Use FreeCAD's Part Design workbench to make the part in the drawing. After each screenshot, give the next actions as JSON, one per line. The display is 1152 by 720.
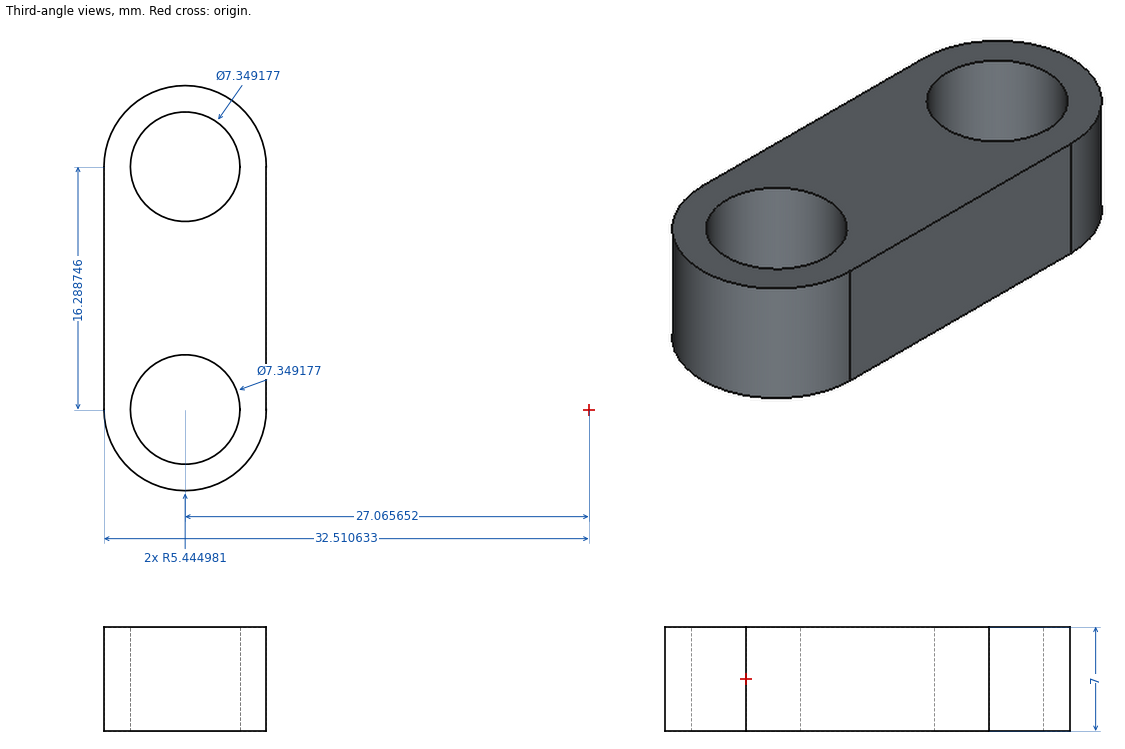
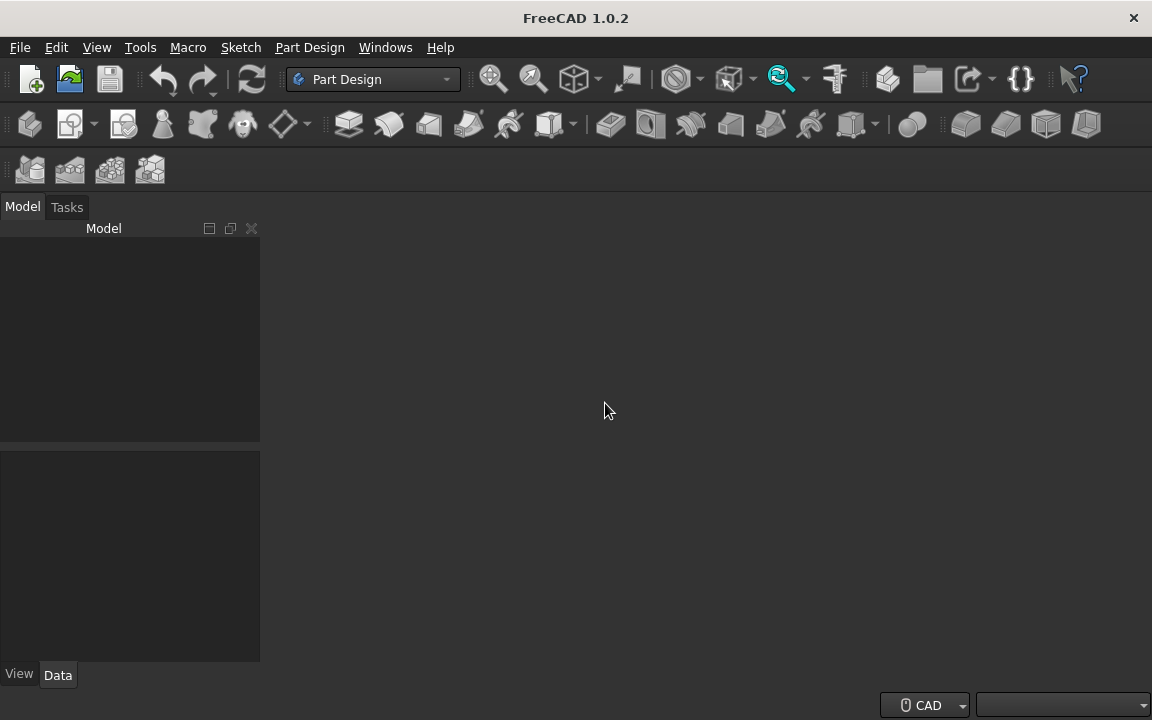
{"action": "left_click", "coordinate": [30, 80]}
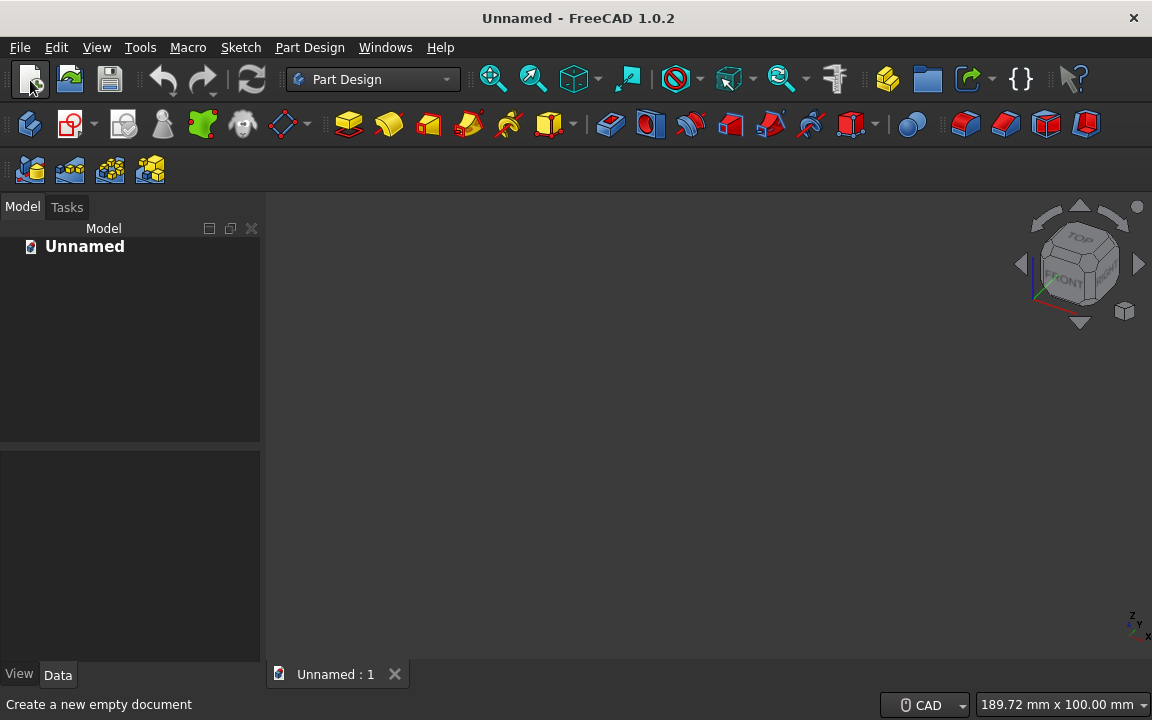
{"action": "left_click", "coordinate": [70, 124]}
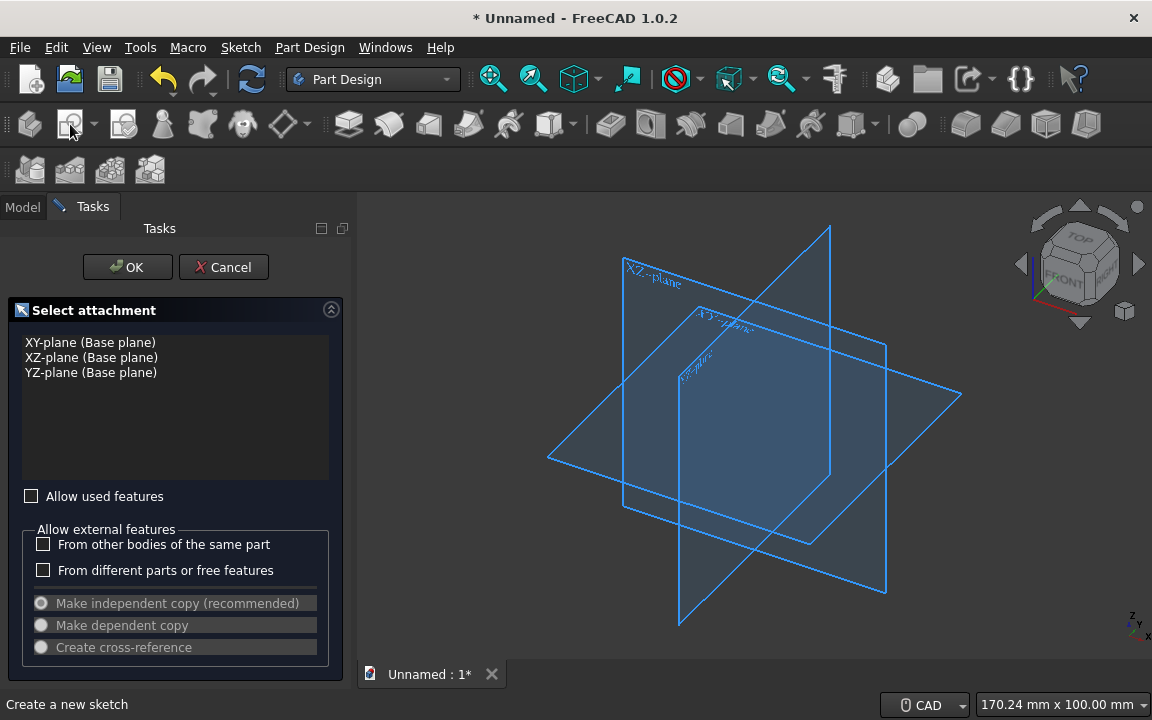
{"action": "left_click", "coordinate": [82, 342]}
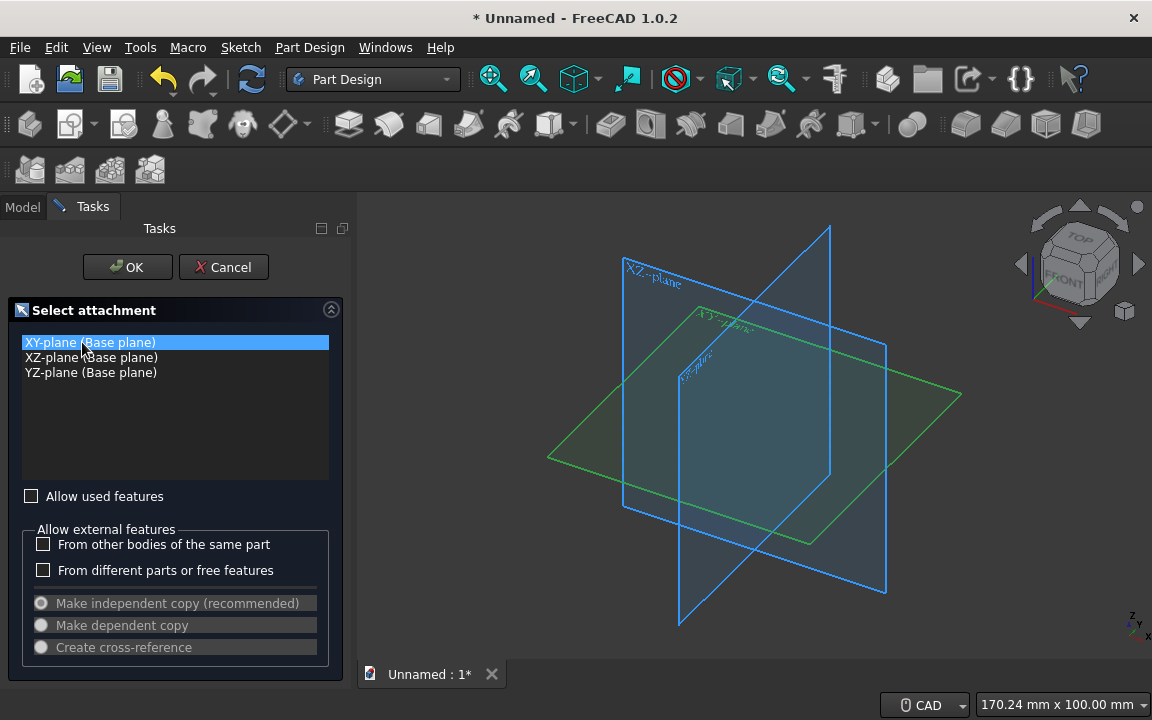
{"action": "left_click", "coordinate": [128, 267]}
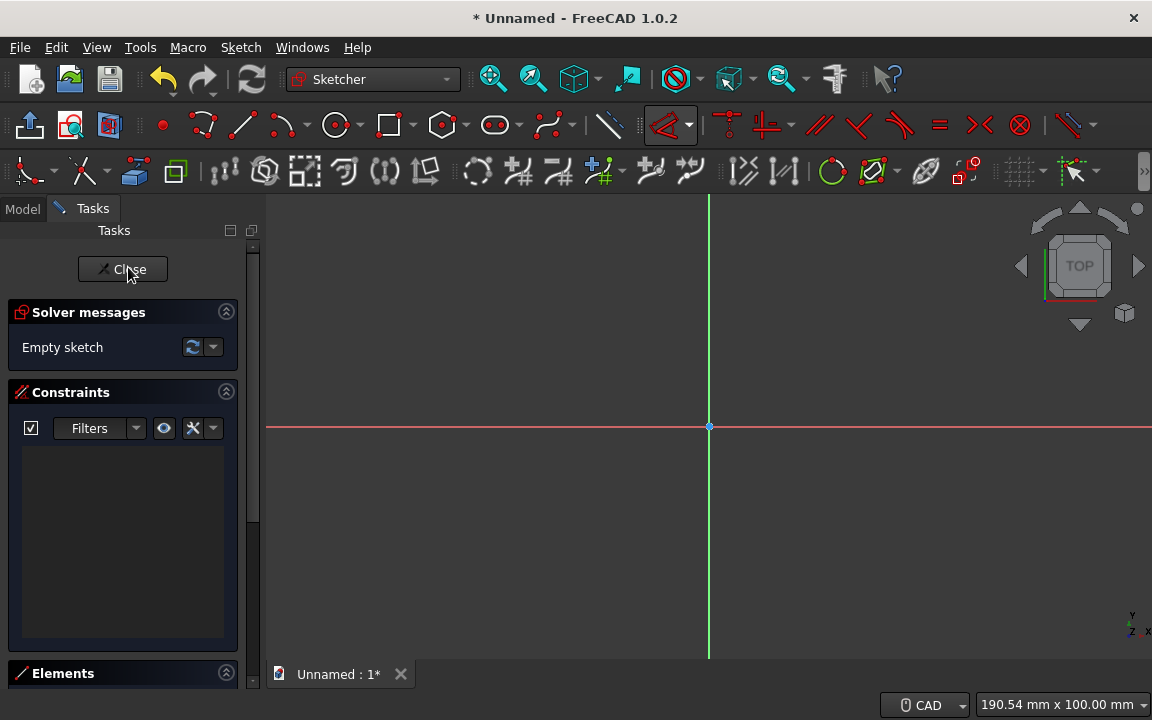
{"action": "scroll", "coordinate": [628, 358], "scroll_direction": "up", "scroll_amount": 4}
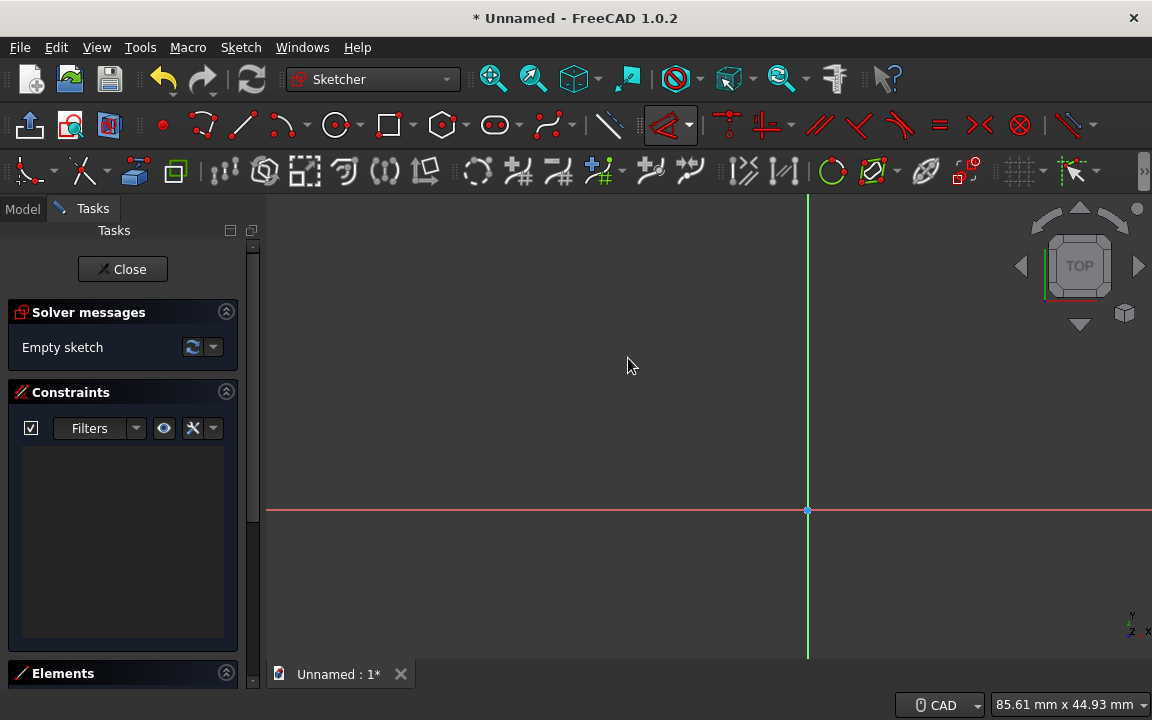
{"action": "left_click", "coordinate": [496, 126]}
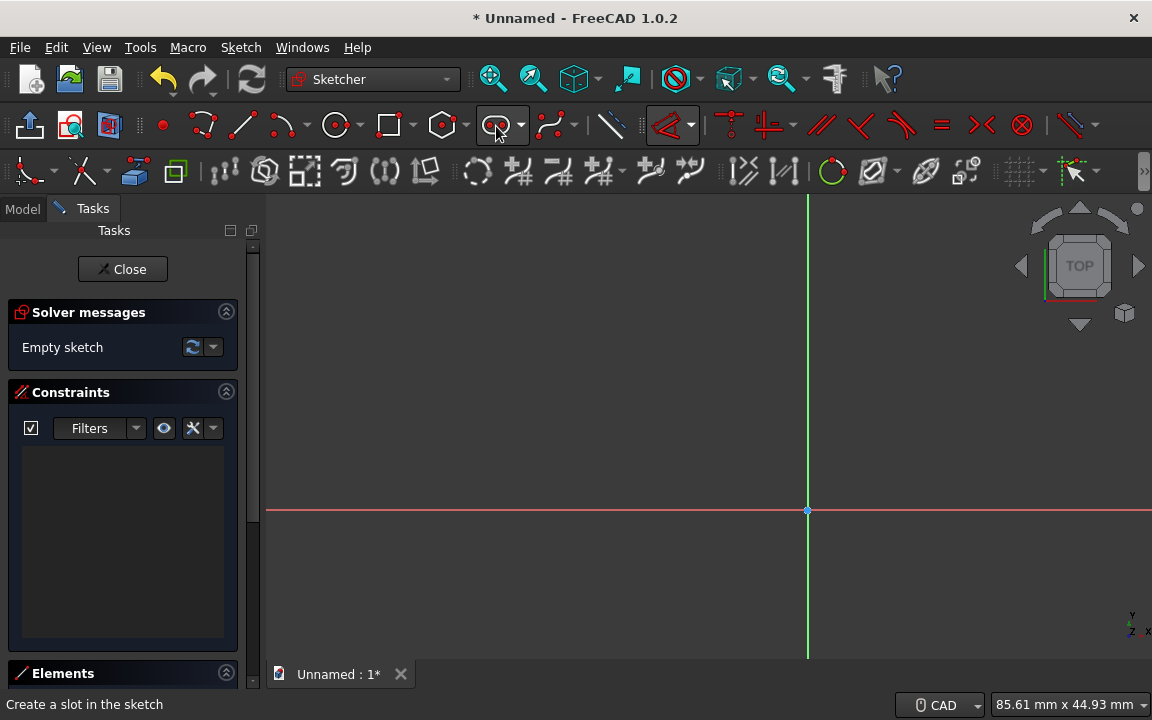
{"action": "left_click", "coordinate": [528, 510]}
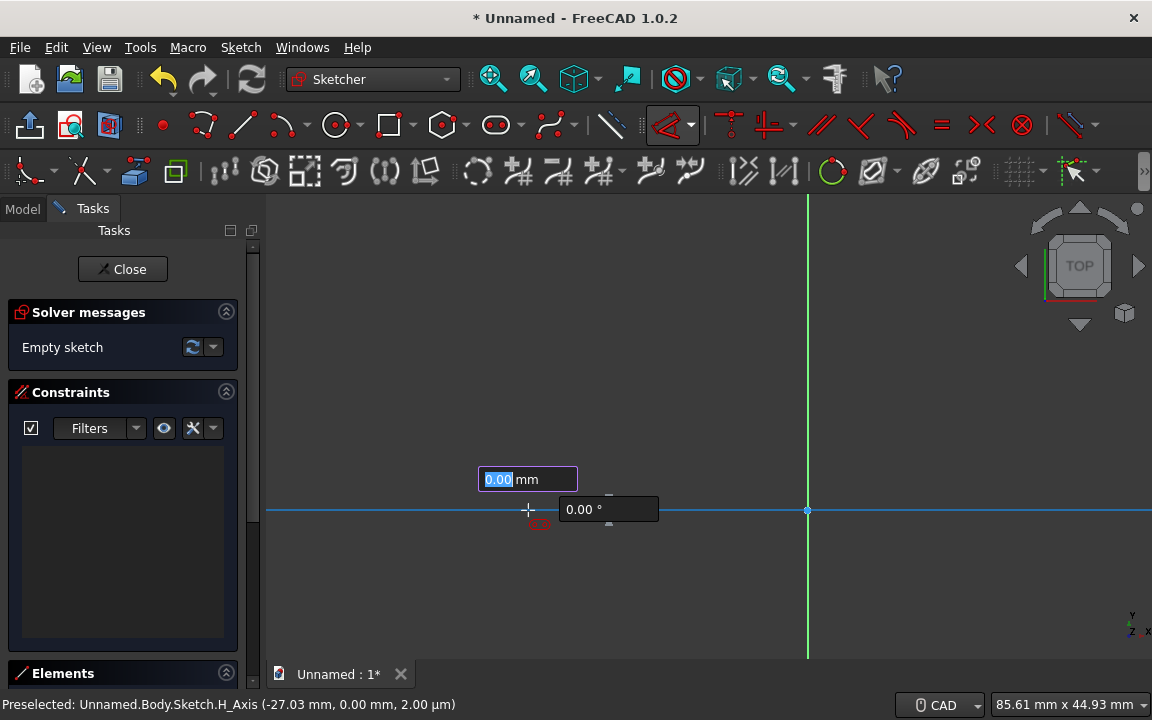
{"action": "left_click", "coordinate": [528, 341]}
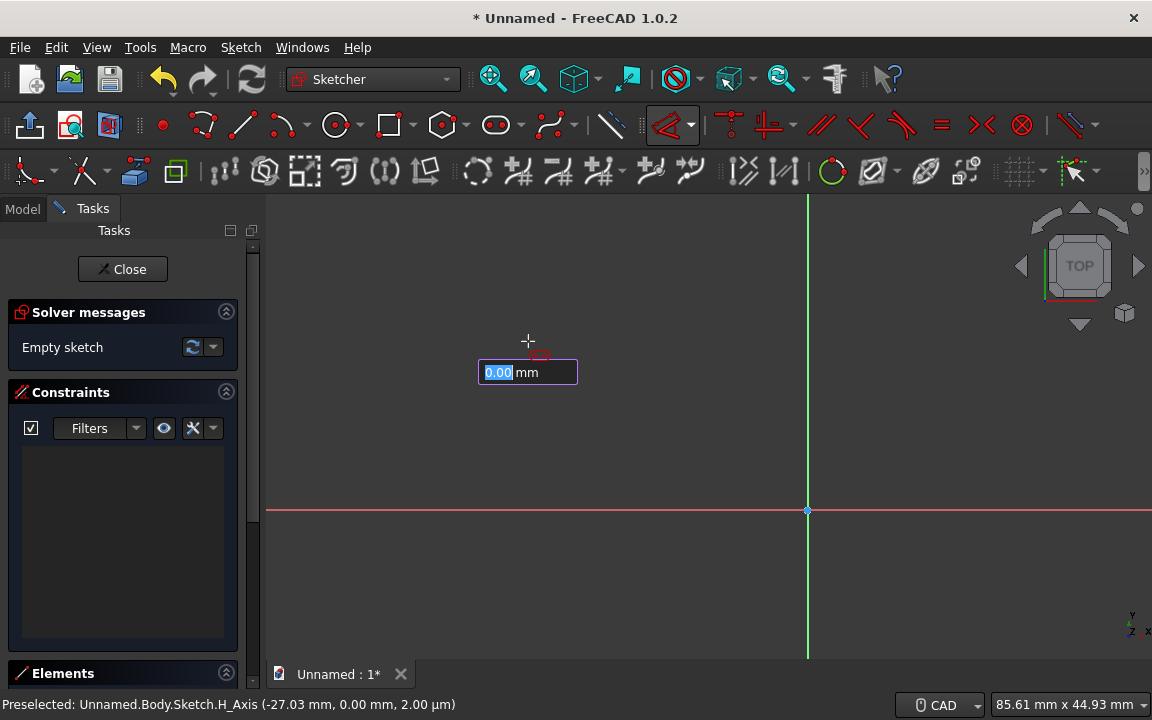
{"action": "left_click", "coordinate": [471, 426]}
{"action": "key", "text": "Escape"}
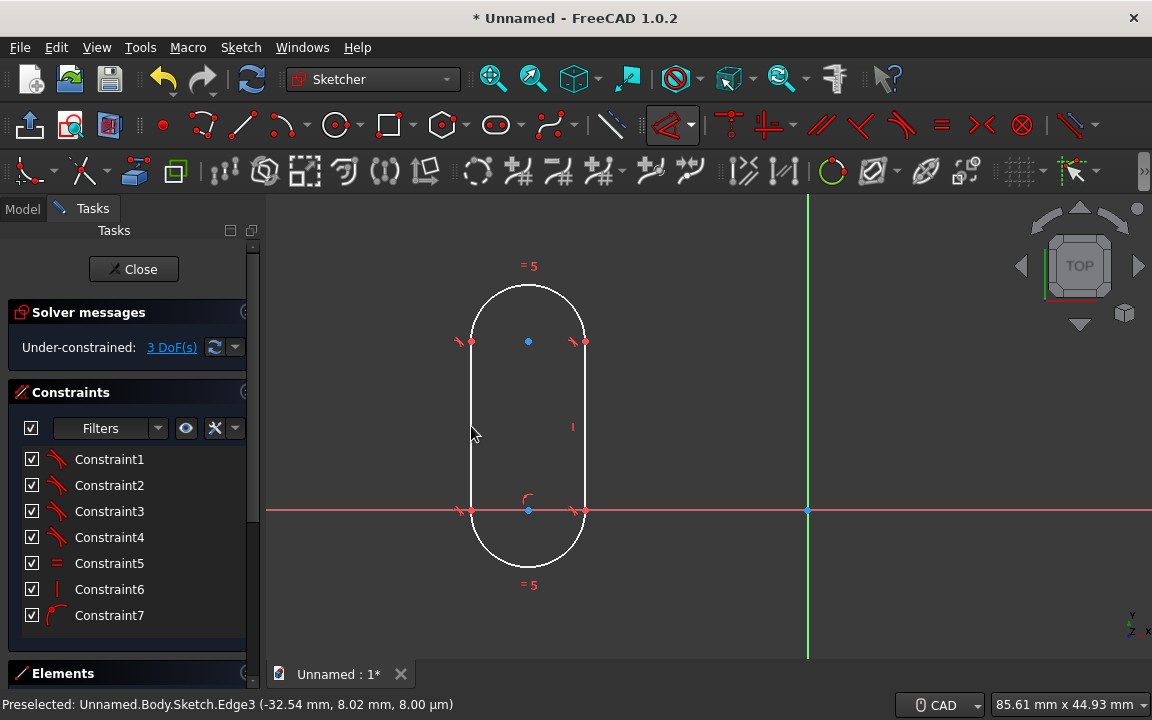
{"action": "key", "text": "d"}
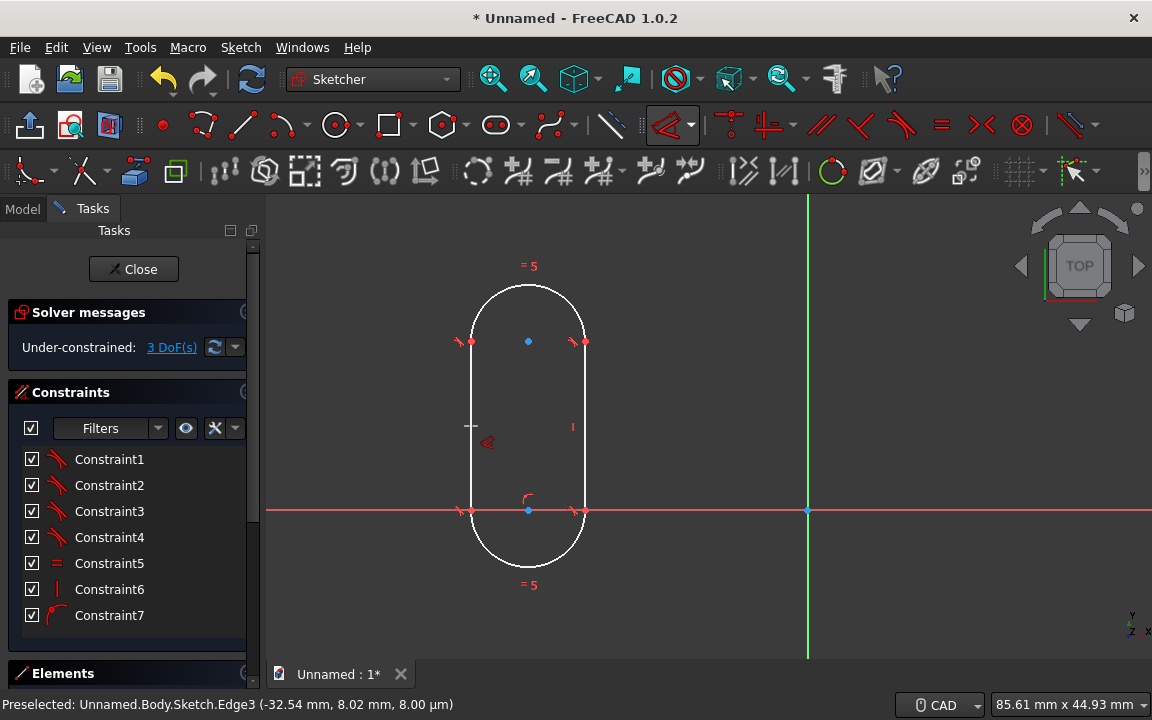
{"action": "left_click", "coordinate": [494, 556]}
{"action": "left_click", "coordinate": [475, 582]}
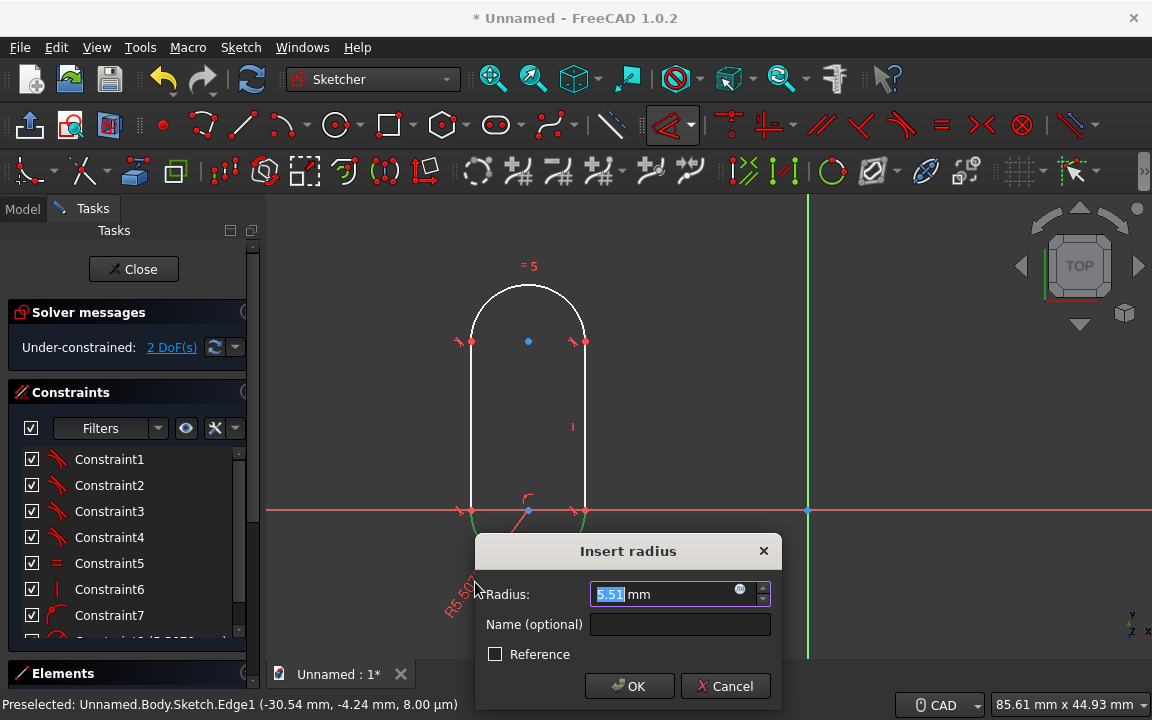
{"action": "type", "text": "5.444981"}
{"action": "key", "text": "Return"}